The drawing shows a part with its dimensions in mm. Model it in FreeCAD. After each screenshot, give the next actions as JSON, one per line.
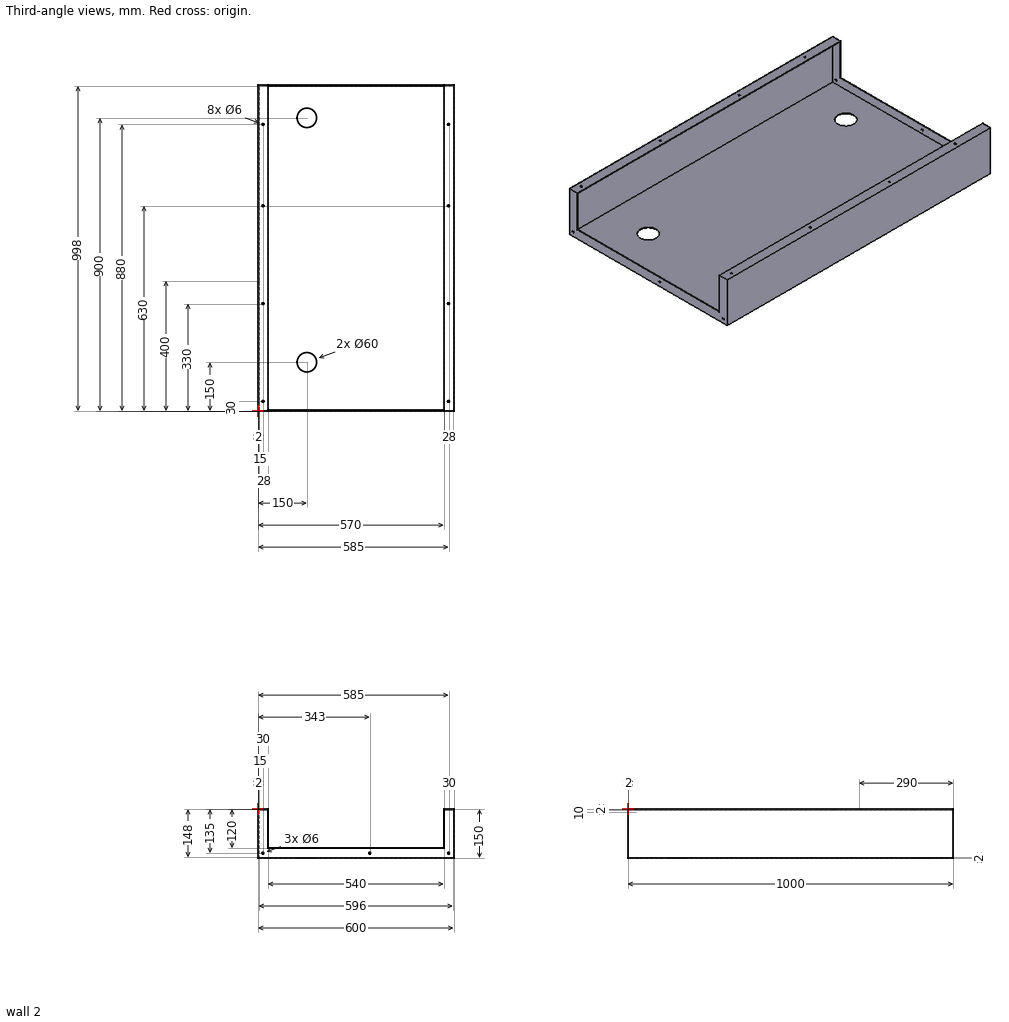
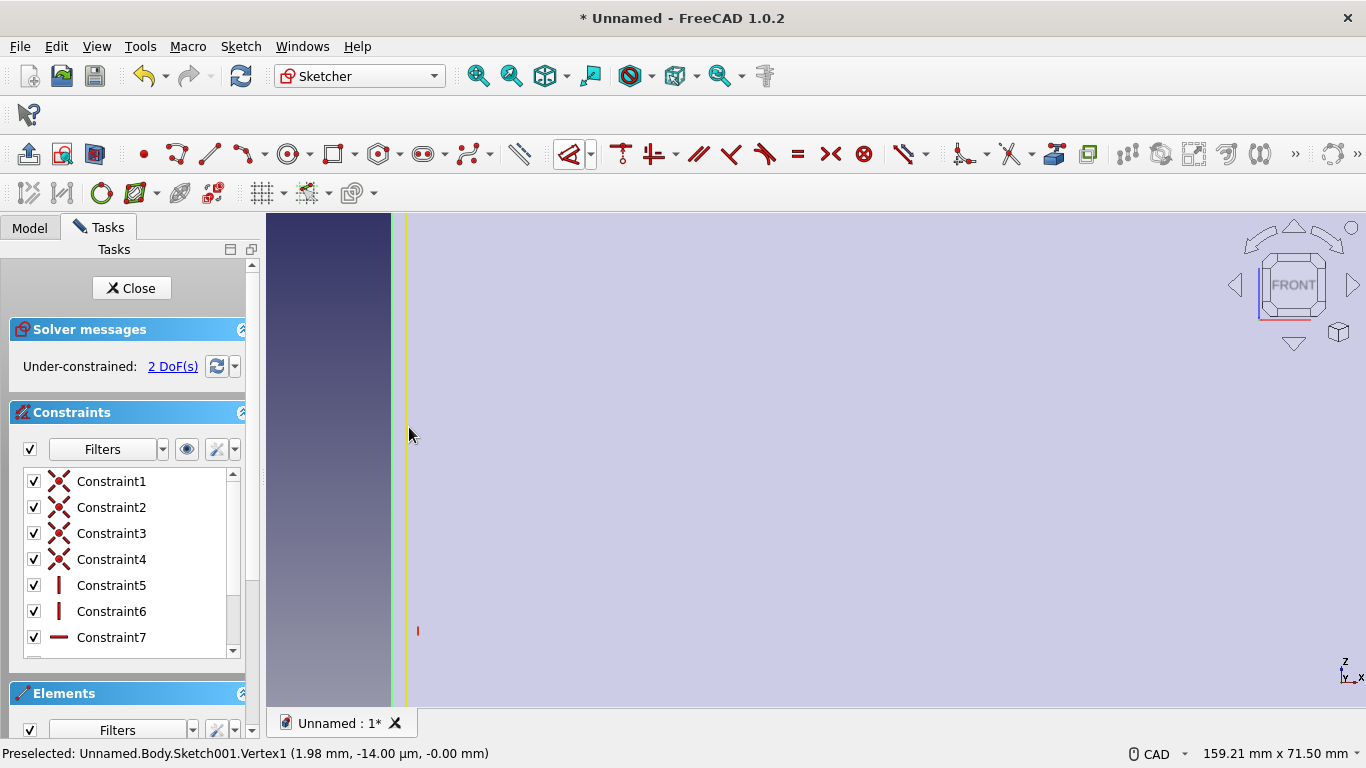
{"action": "left_click", "coordinate": [406, 425]}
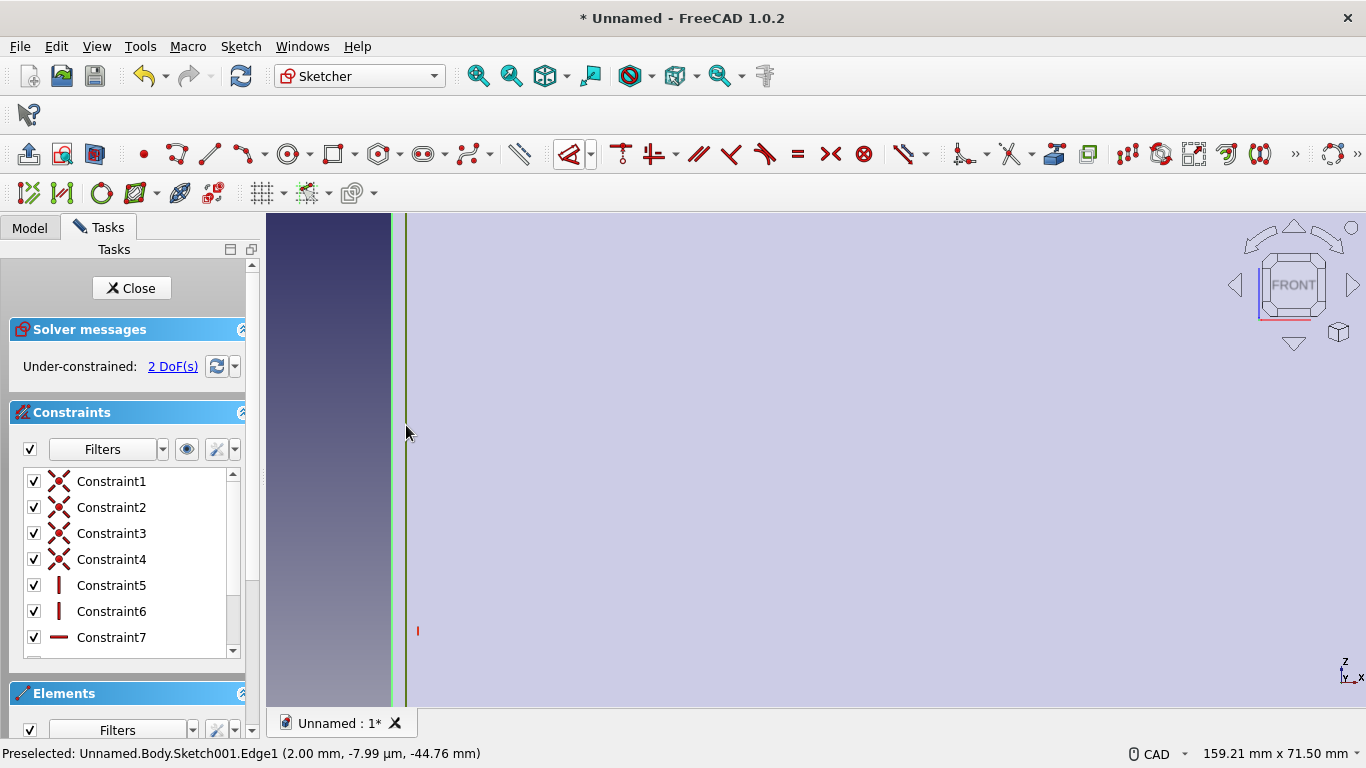
{"action": "key", "text": "i"}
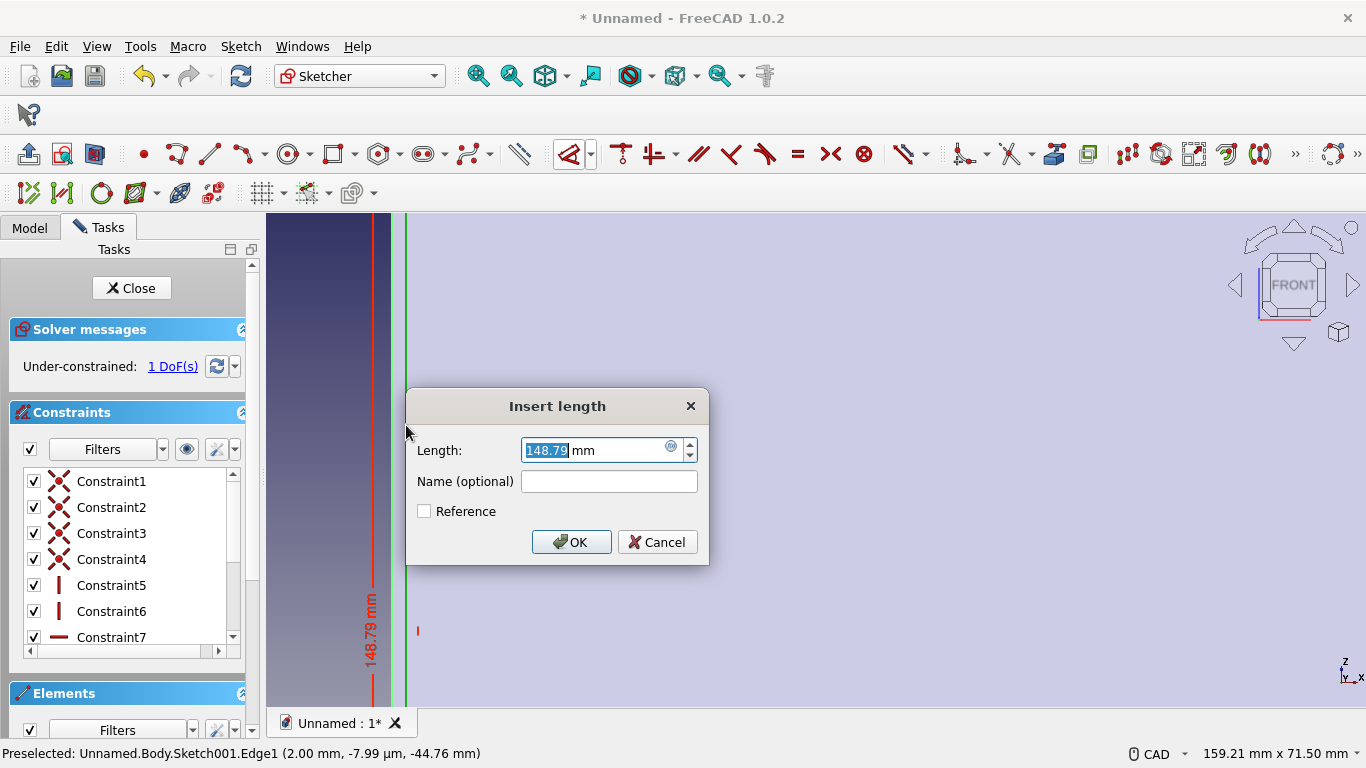
{"action": "type", "text": "148"}
{"action": "key", "text": "Return"}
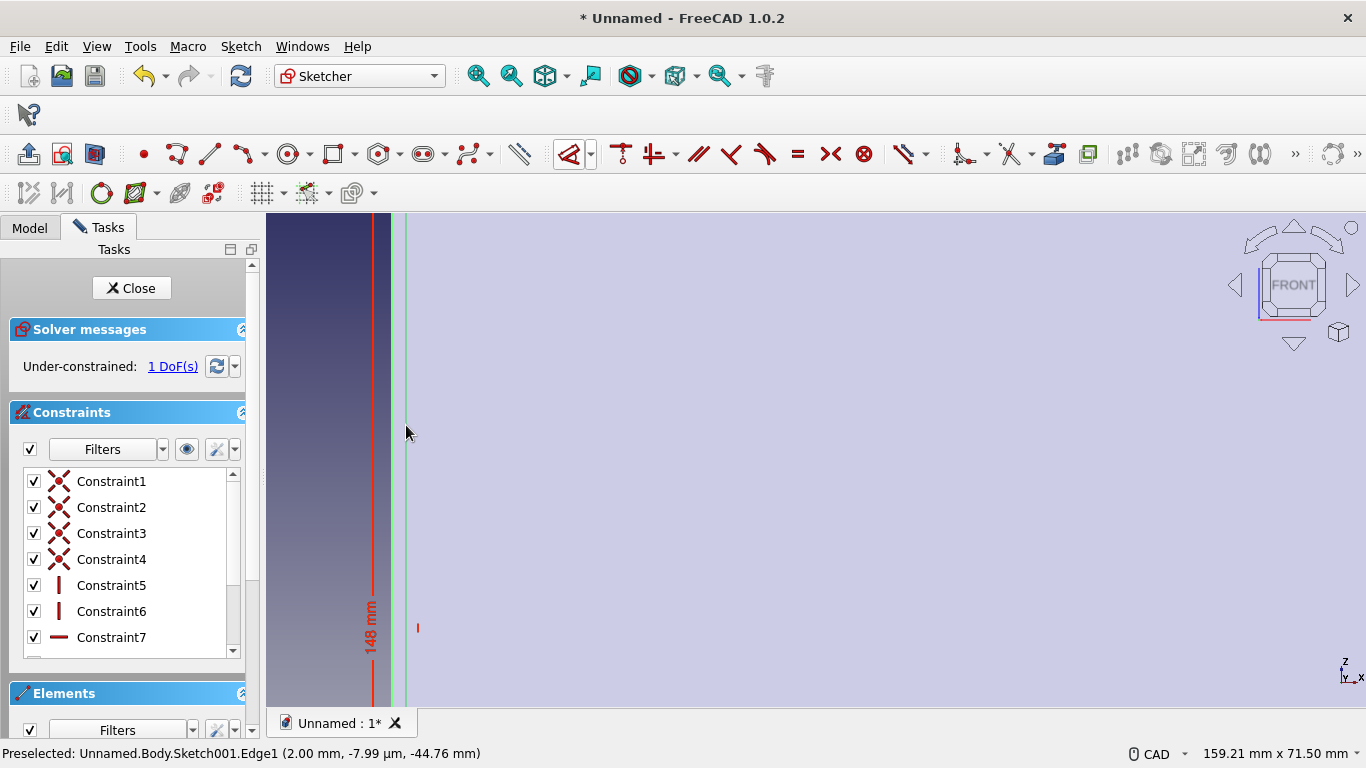
{"action": "scroll", "coordinate": [409, 427], "scroll_direction": "down", "scroll_amount": 9}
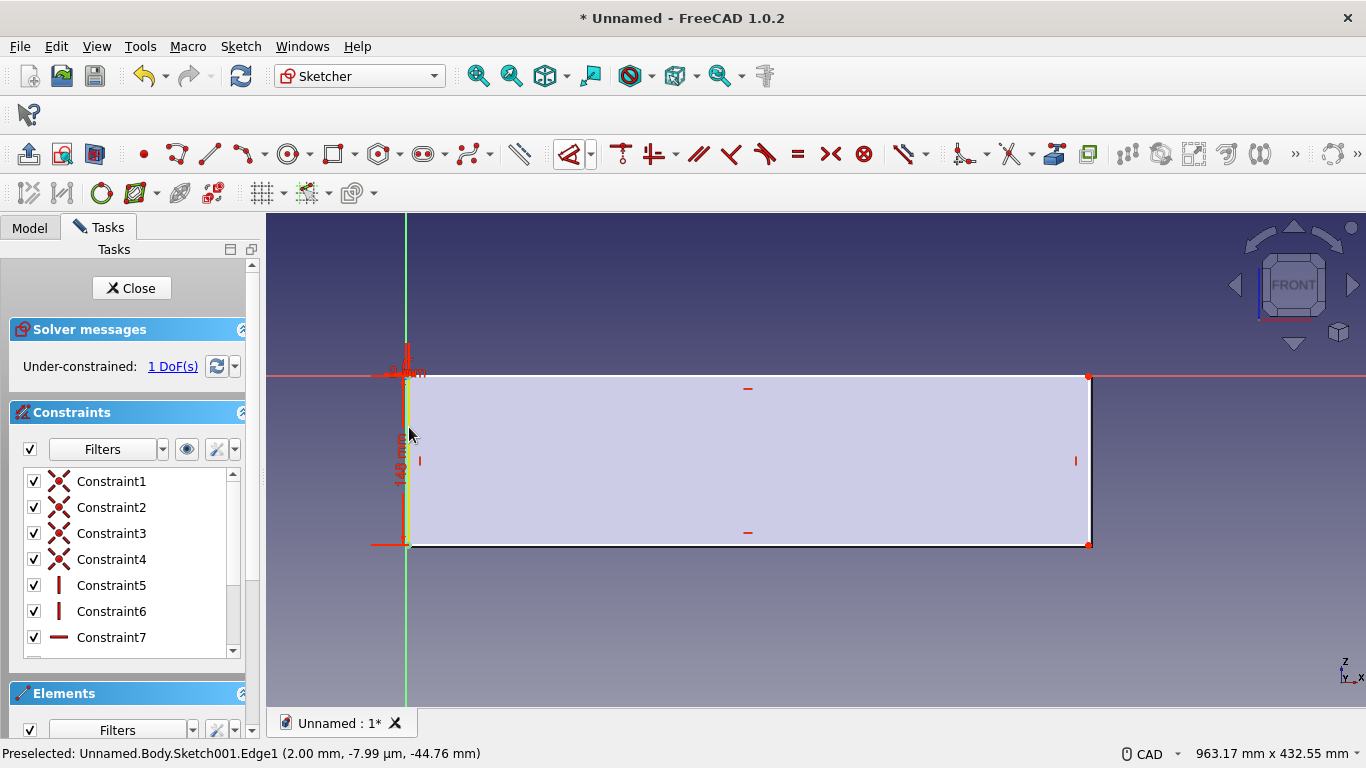
{"action": "left_click", "coordinate": [613, 545]}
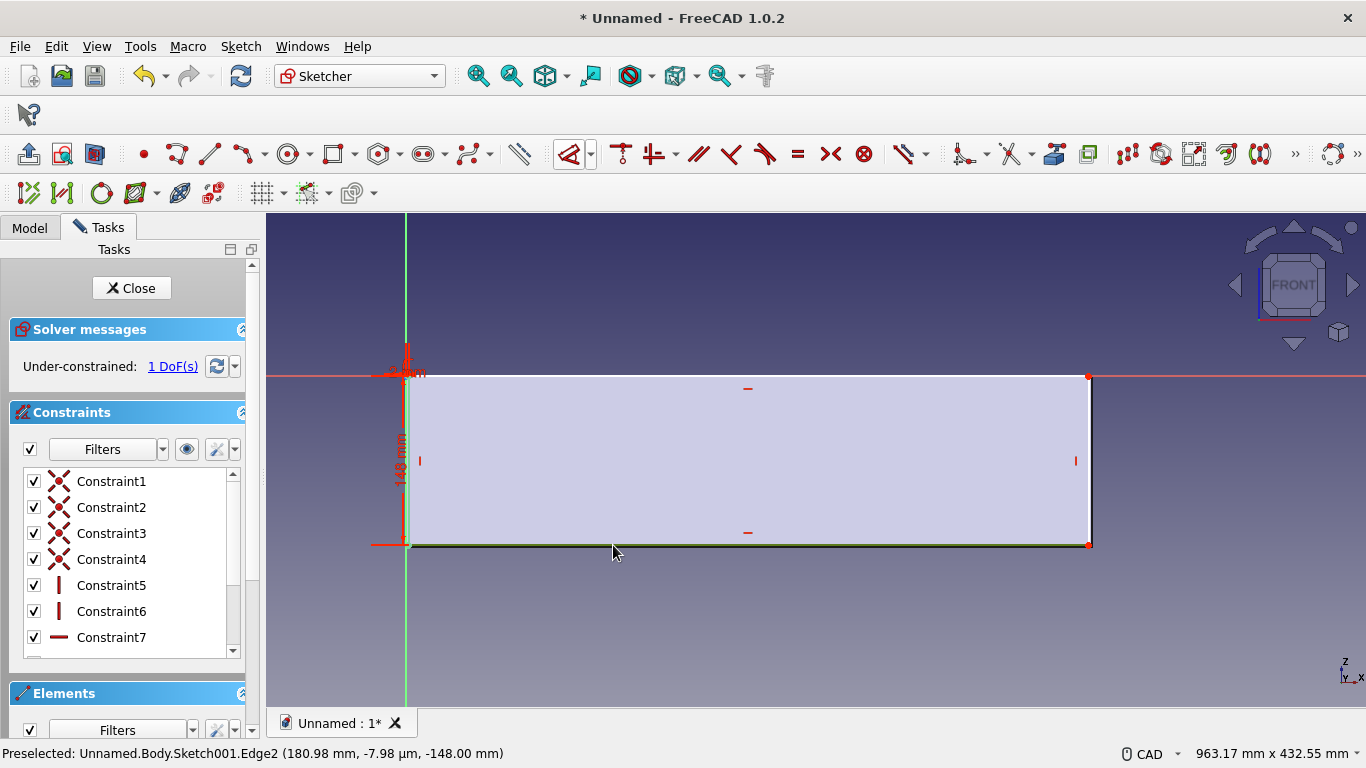
{"action": "key", "text": "l"}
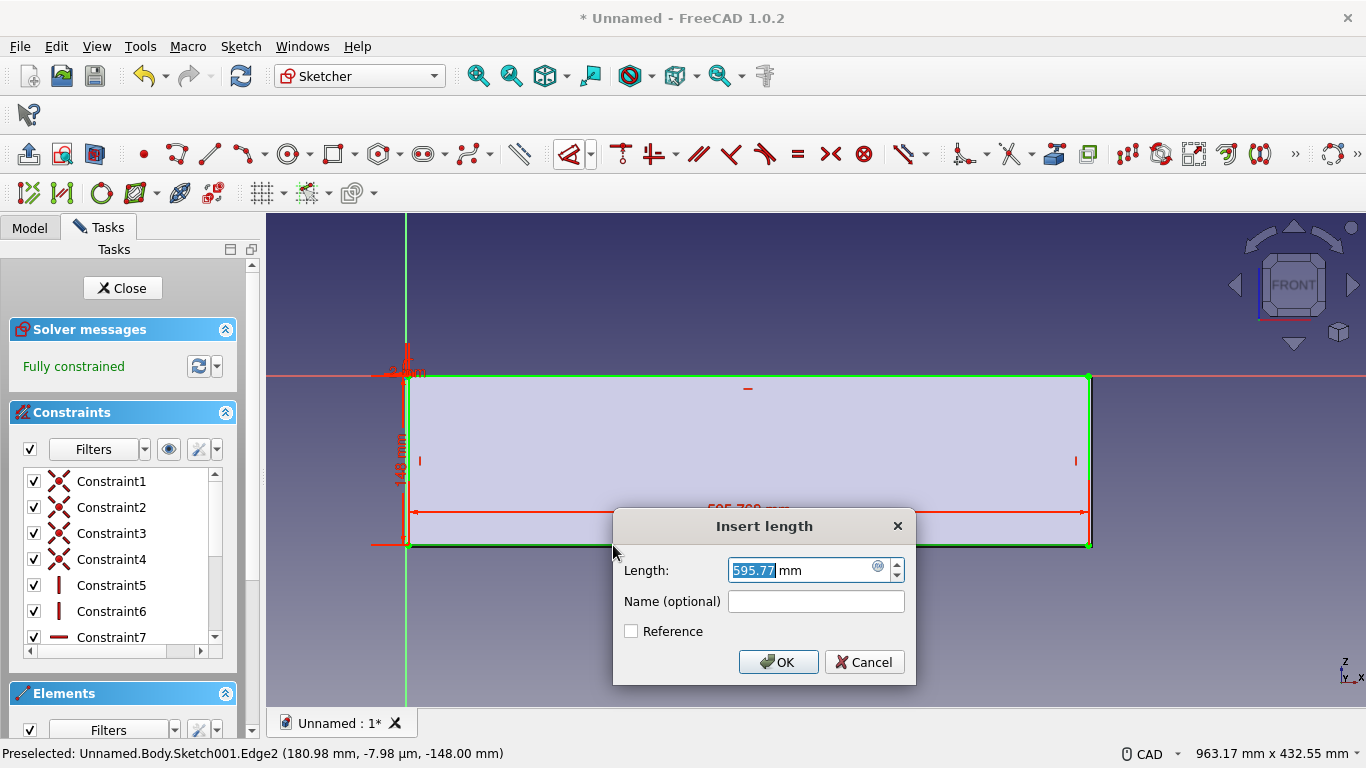
{"action": "type", "text": "596"}
{"action": "key", "text": "Return"}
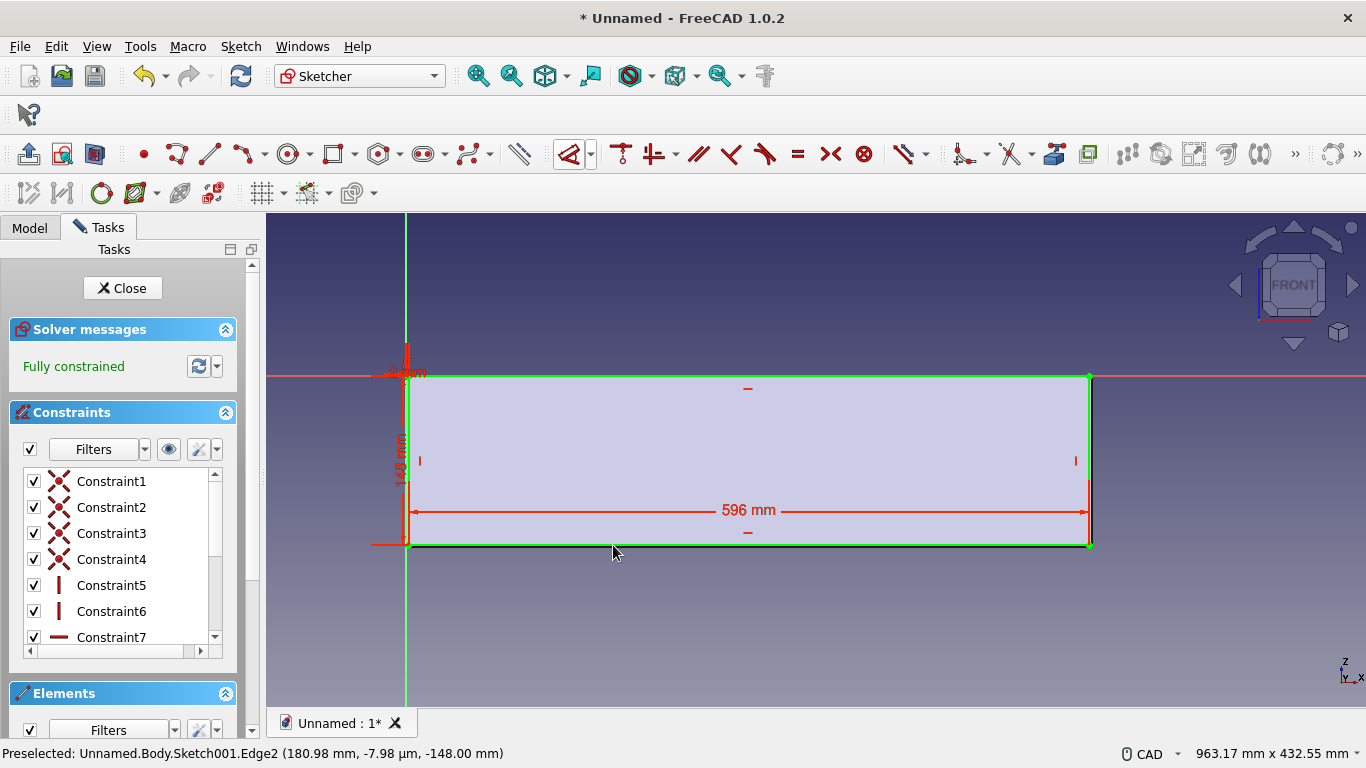
{"action": "left_click", "coordinate": [123, 288]}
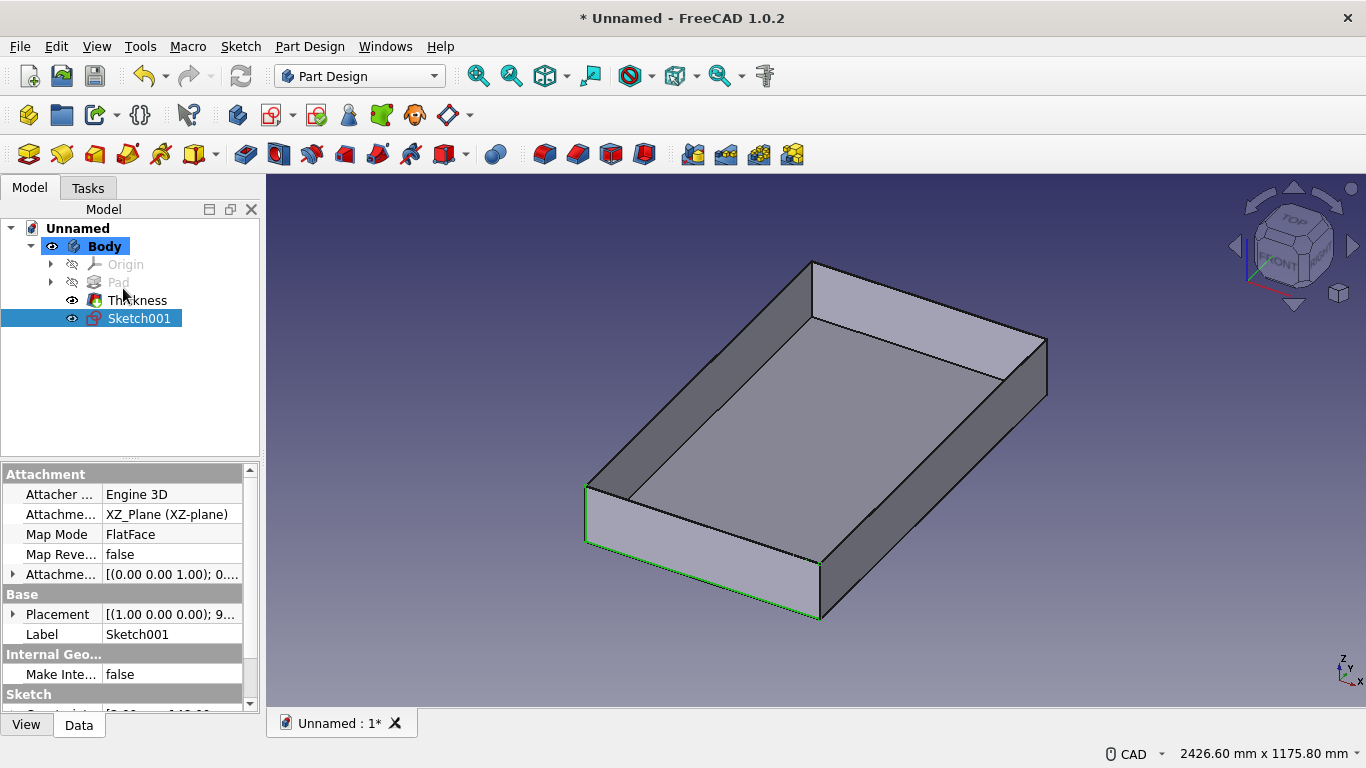
{"action": "left_click", "coordinate": [246, 154]}